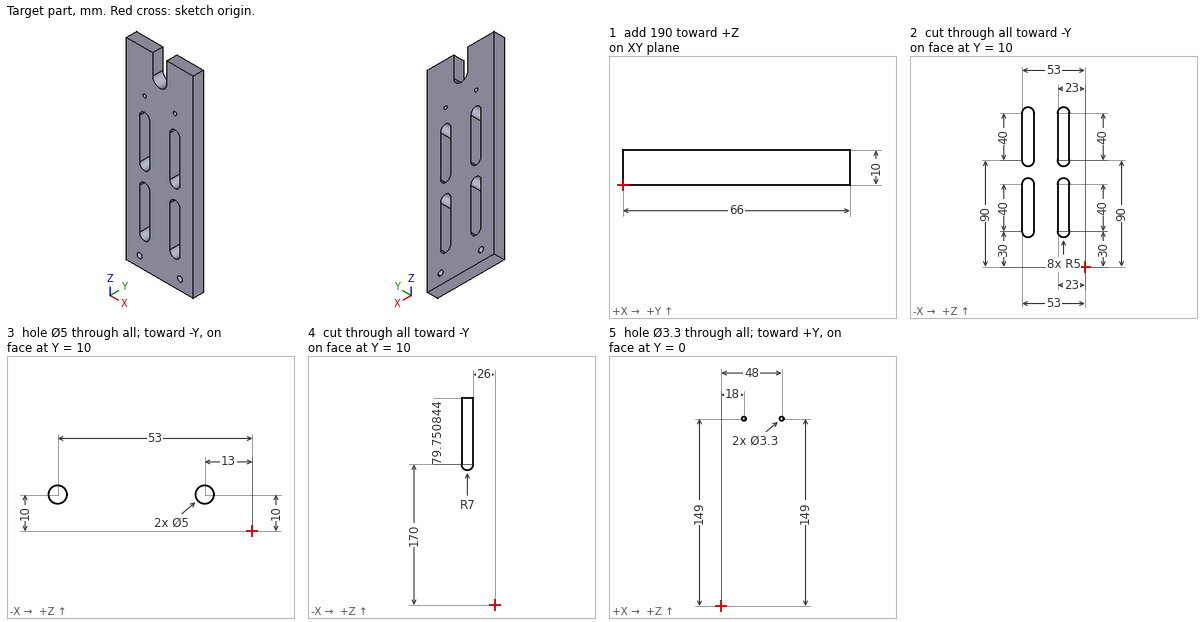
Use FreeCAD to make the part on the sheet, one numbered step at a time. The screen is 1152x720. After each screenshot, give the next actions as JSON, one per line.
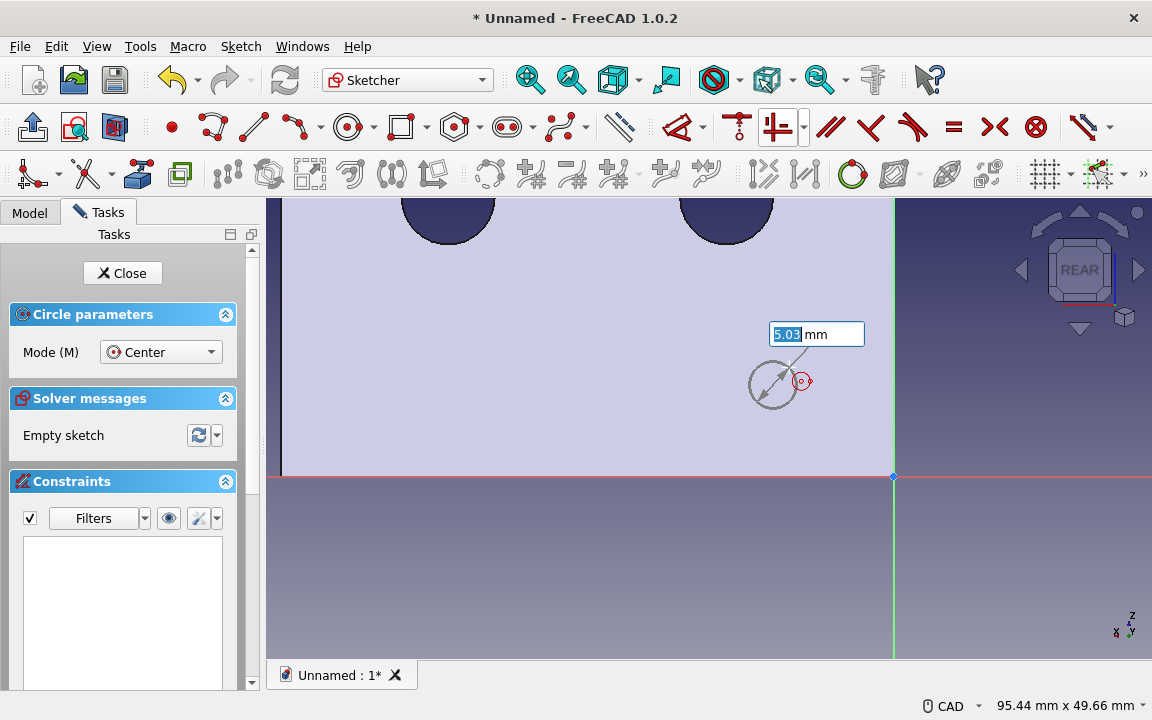
{"action": "type", "text": "5"}
{"action": "key", "text": "Return"}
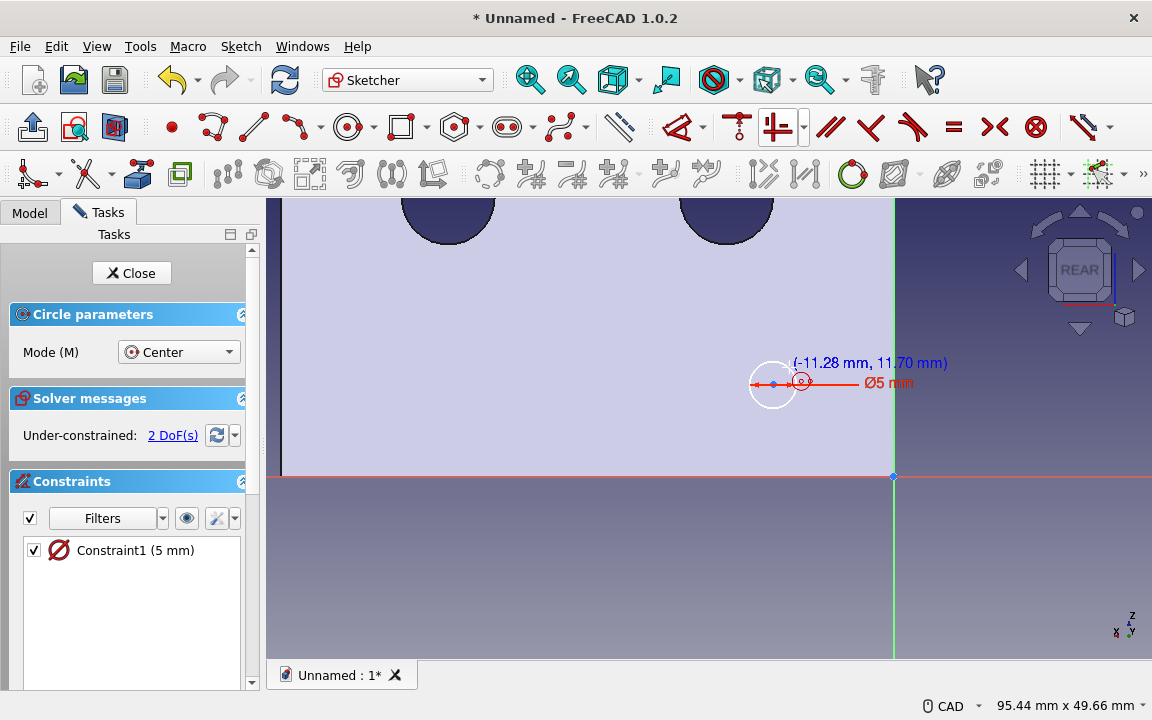
{"action": "left_click", "coordinate": [402, 384]}
{"action": "mouse_move", "coordinate": [418, 367]}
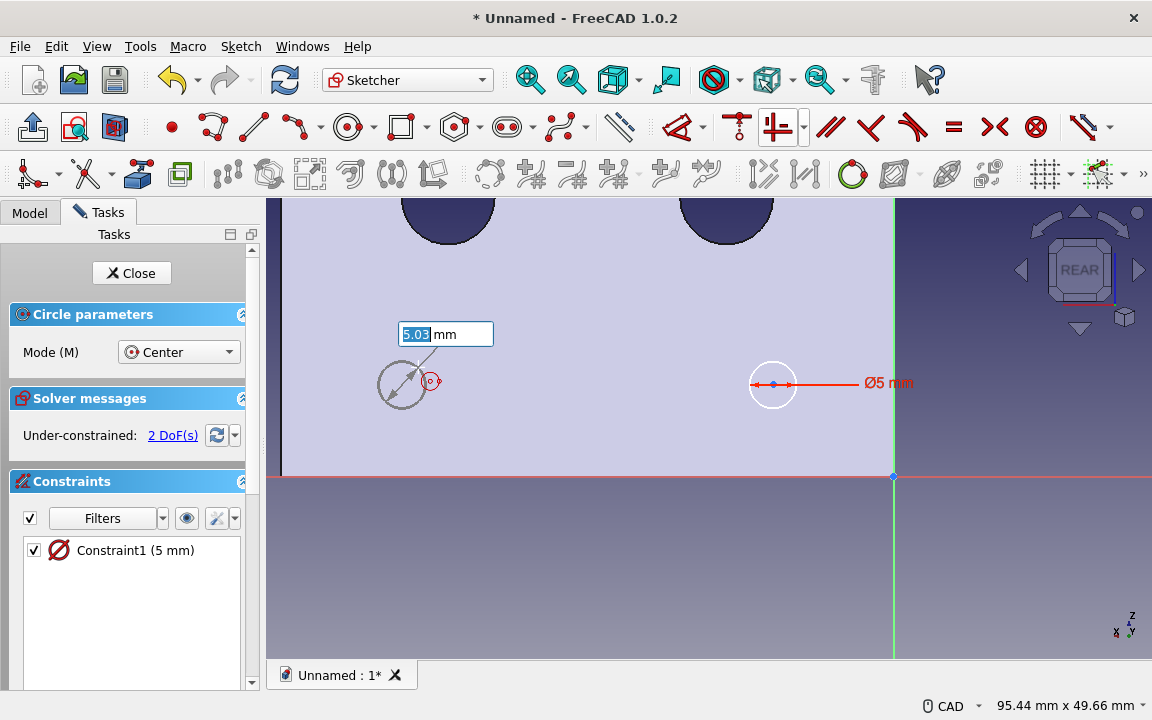
{"action": "type", "text": "5"}
{"action": "key", "text": "Return"}
{"action": "key", "text": "Escape"}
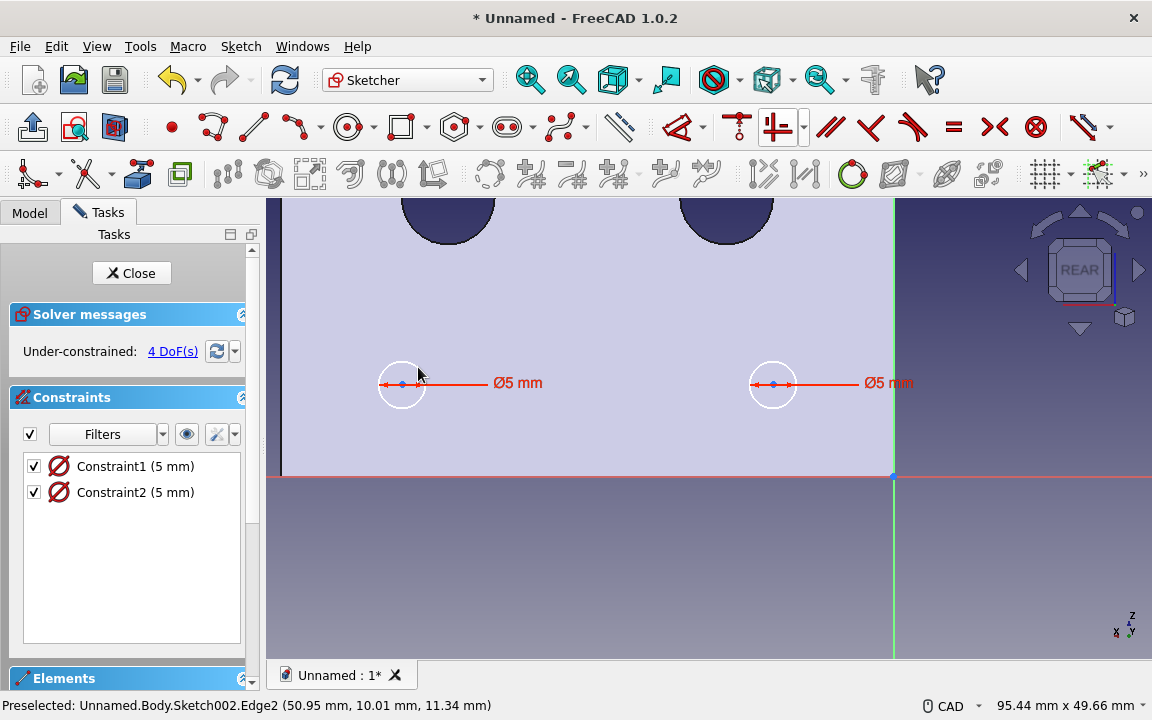
{"action": "left_click", "coordinate": [676, 128]}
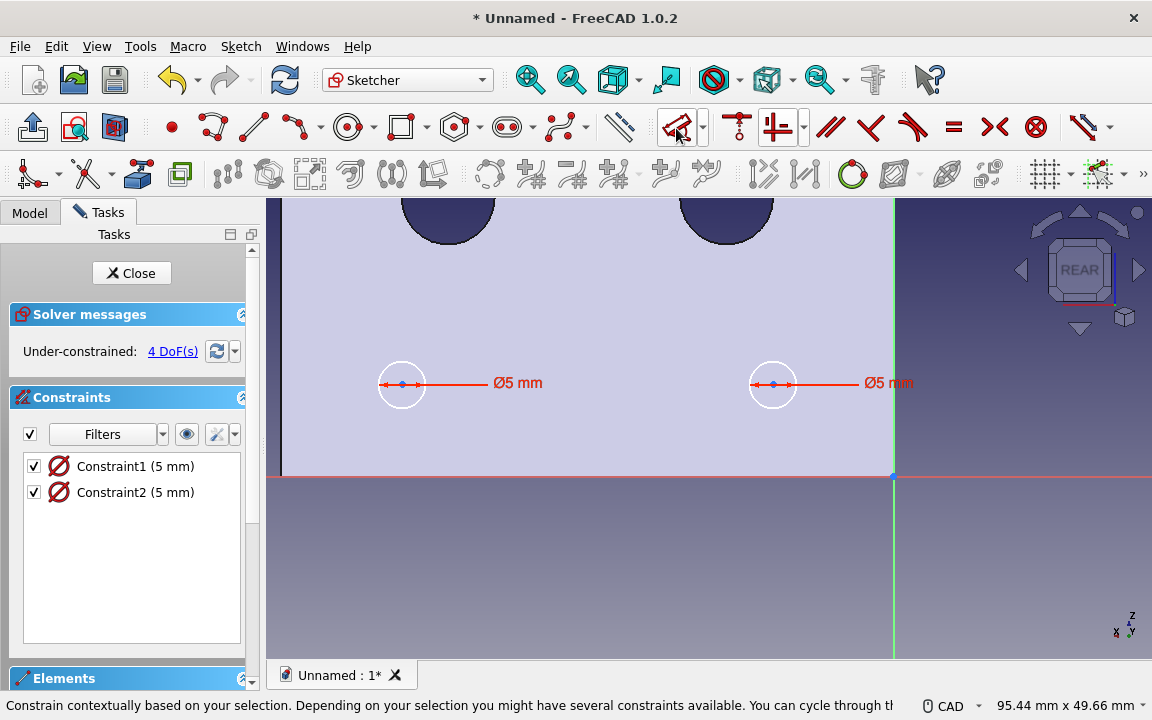
{"action": "left_click", "coordinate": [773, 385]}
{"action": "left_click", "coordinate": [833, 511]}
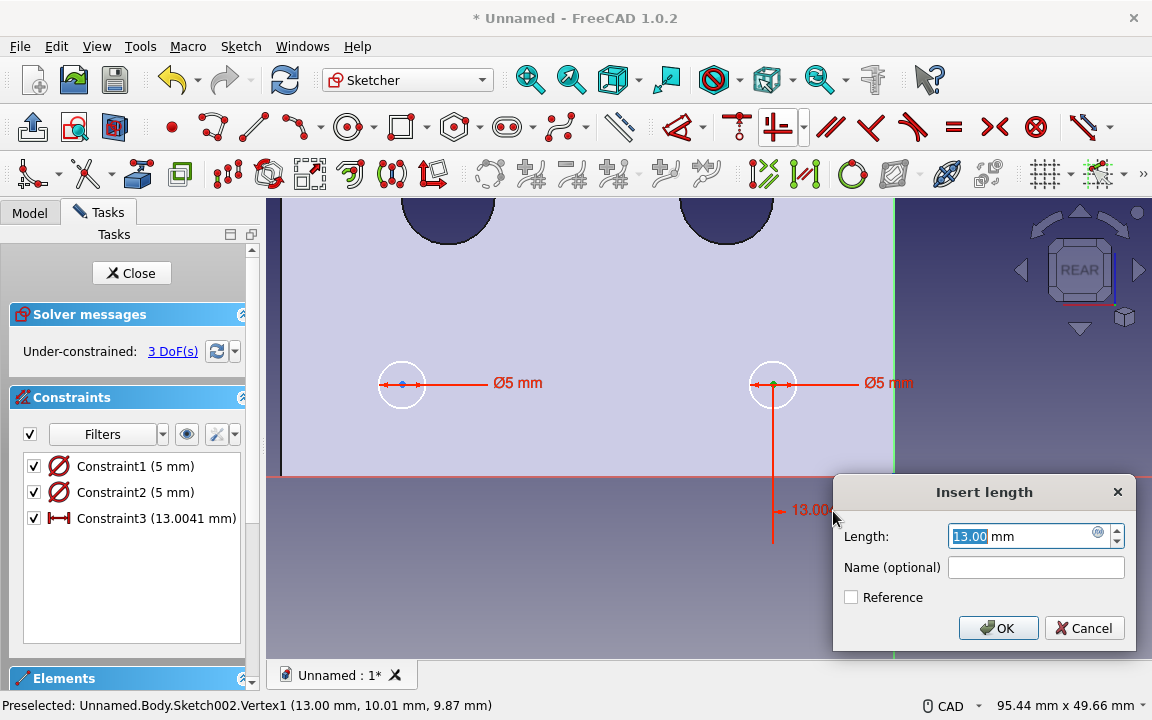
{"action": "type", "text": "13"}
{"action": "key", "text": "Return"}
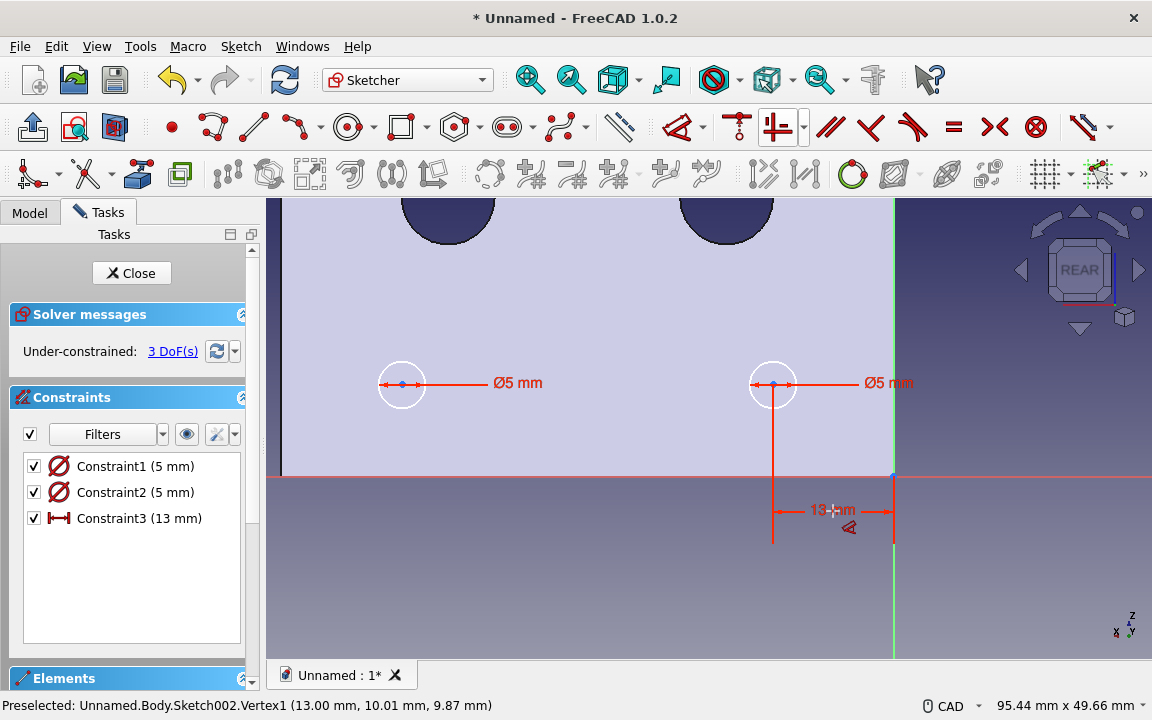
{"action": "left_click", "coordinate": [773, 385]}
{"action": "left_click", "coordinate": [928, 431]}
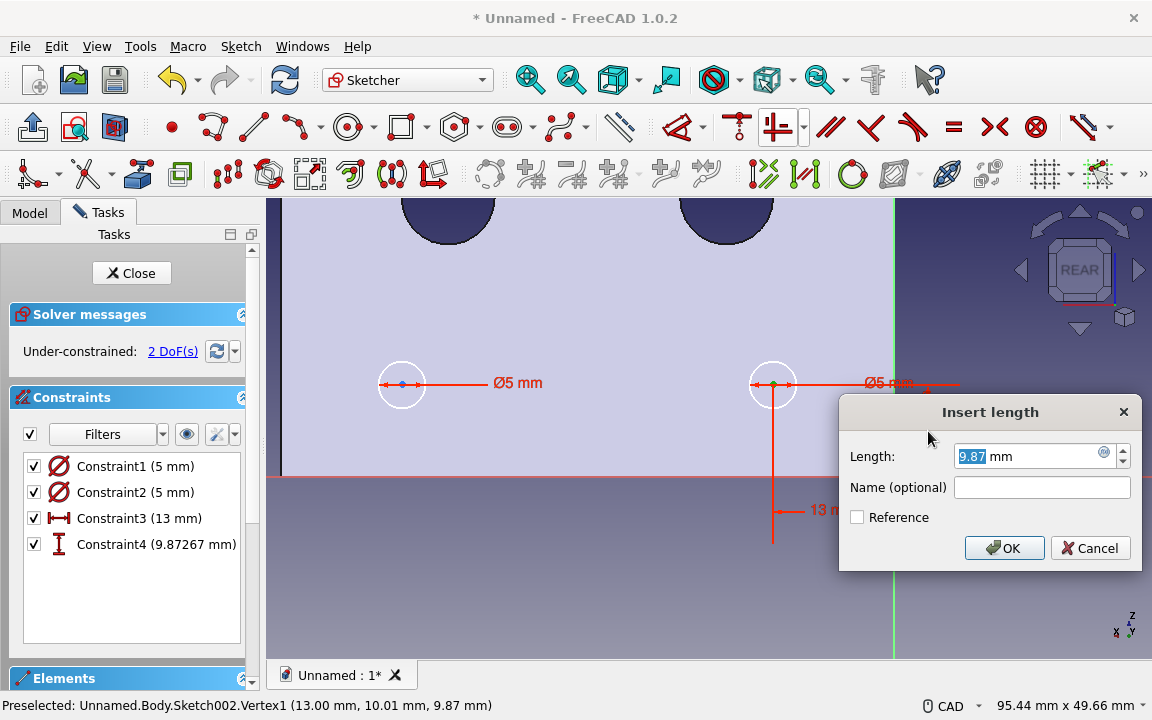
{"action": "type", "text": "10"}
{"action": "key", "text": "Return"}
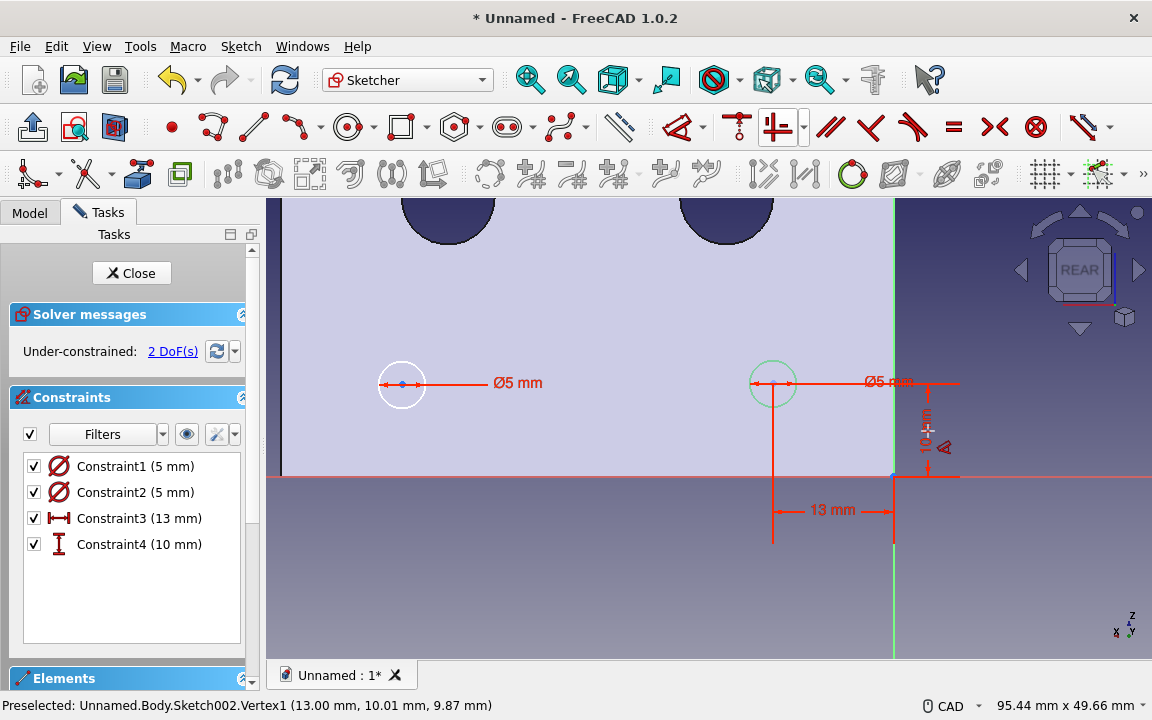
{"action": "left_click", "coordinate": [402, 385]}
{"action": "left_click", "coordinate": [648, 511]}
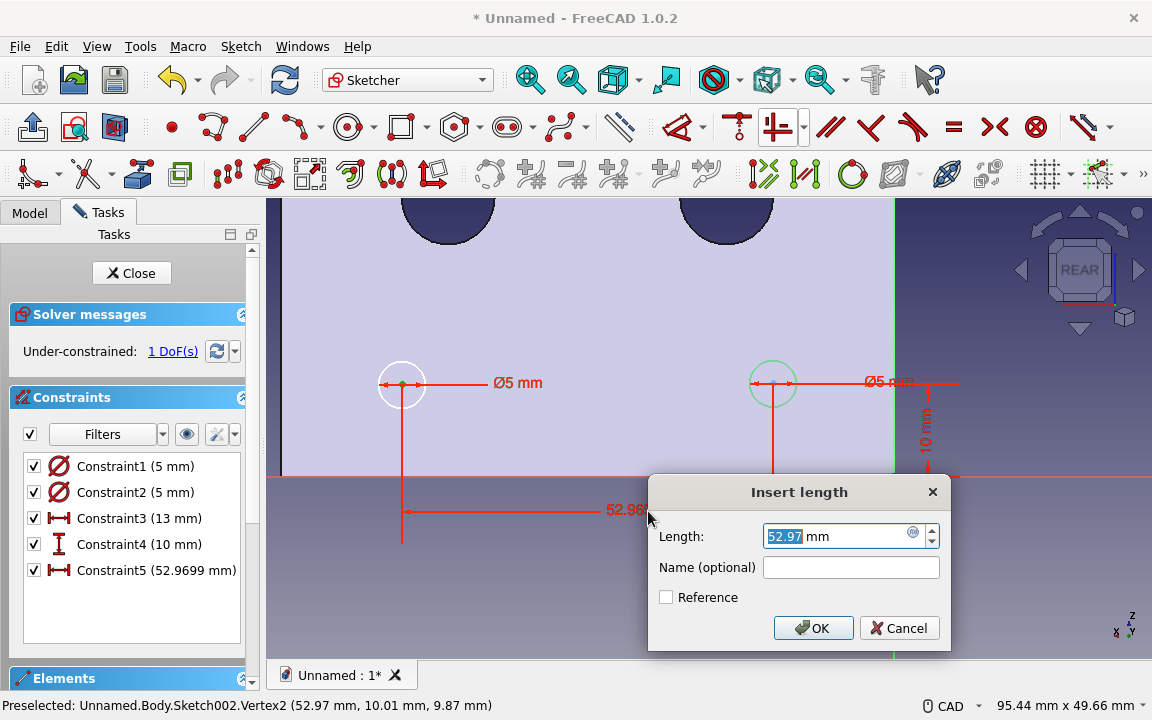
{"action": "type", "text": "53"}
{"action": "key", "text": "Return"}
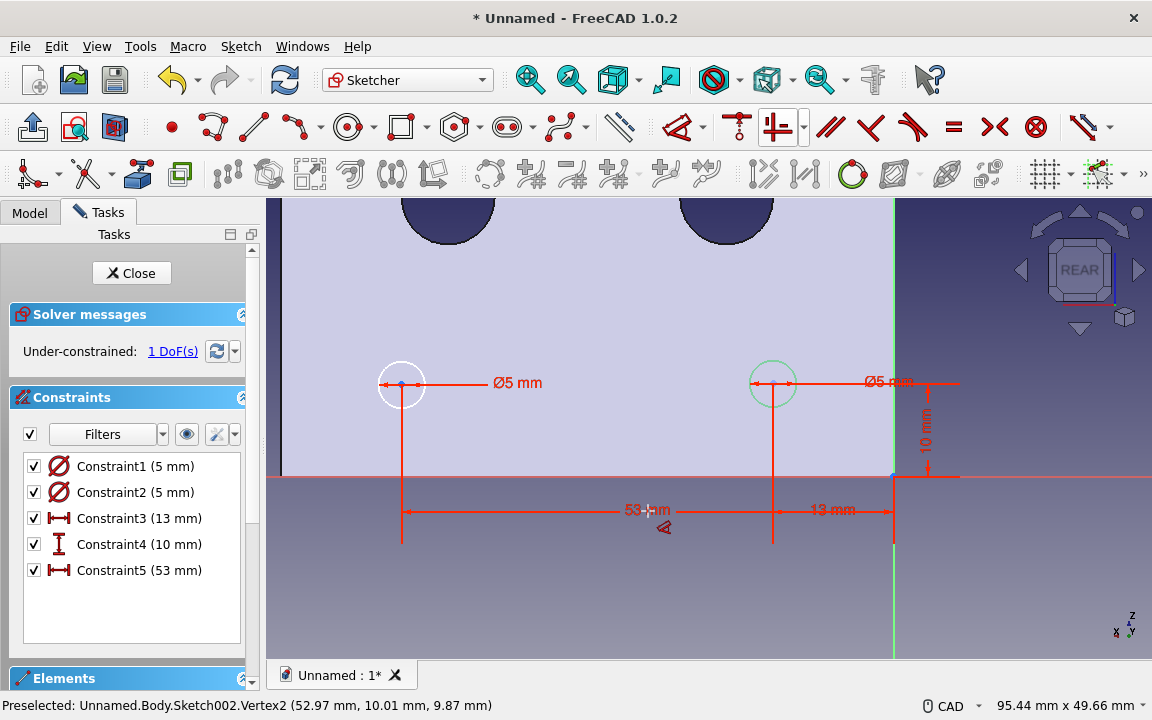
{"action": "left_click", "coordinate": [402, 385]}
{"action": "left_click", "coordinate": [928, 410]}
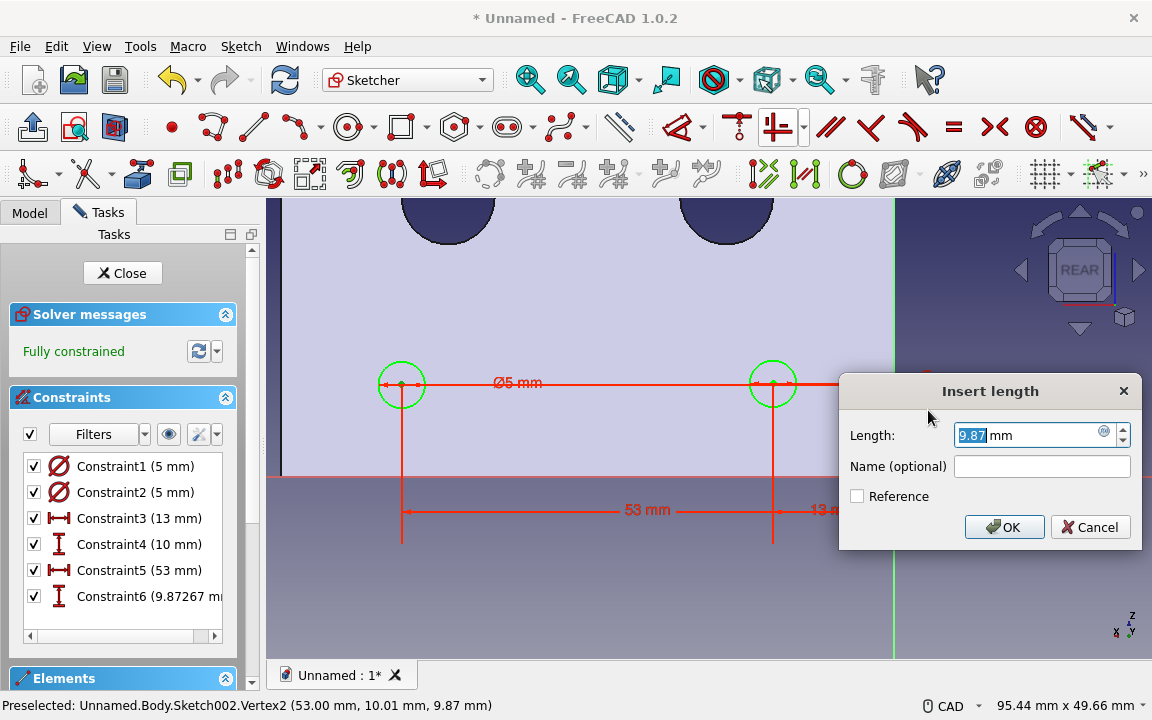
{"action": "type", "text": "10"}
{"action": "key", "text": "Return"}
{"action": "key", "text": "Escape"}